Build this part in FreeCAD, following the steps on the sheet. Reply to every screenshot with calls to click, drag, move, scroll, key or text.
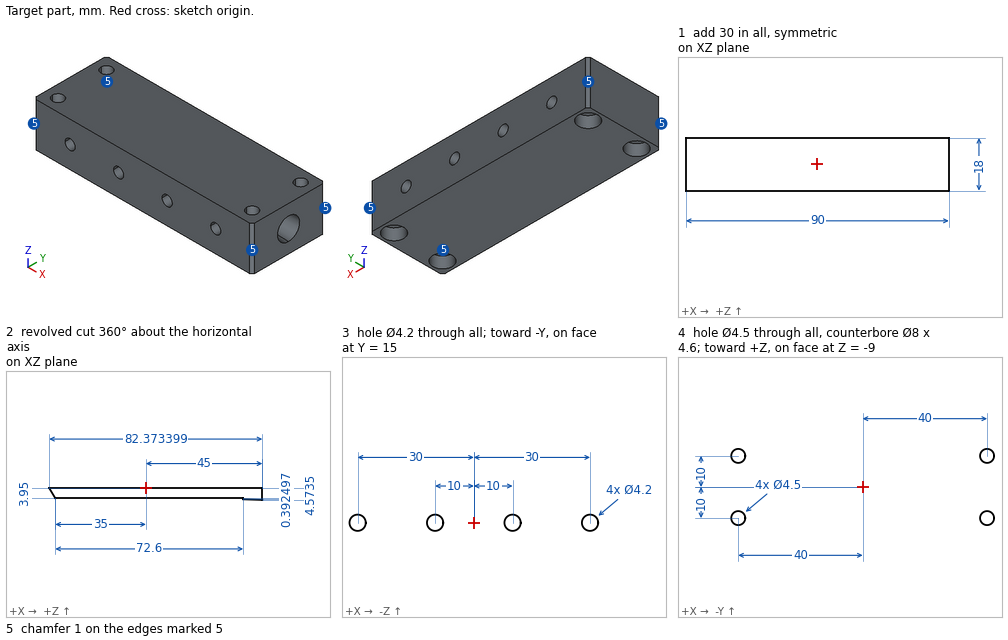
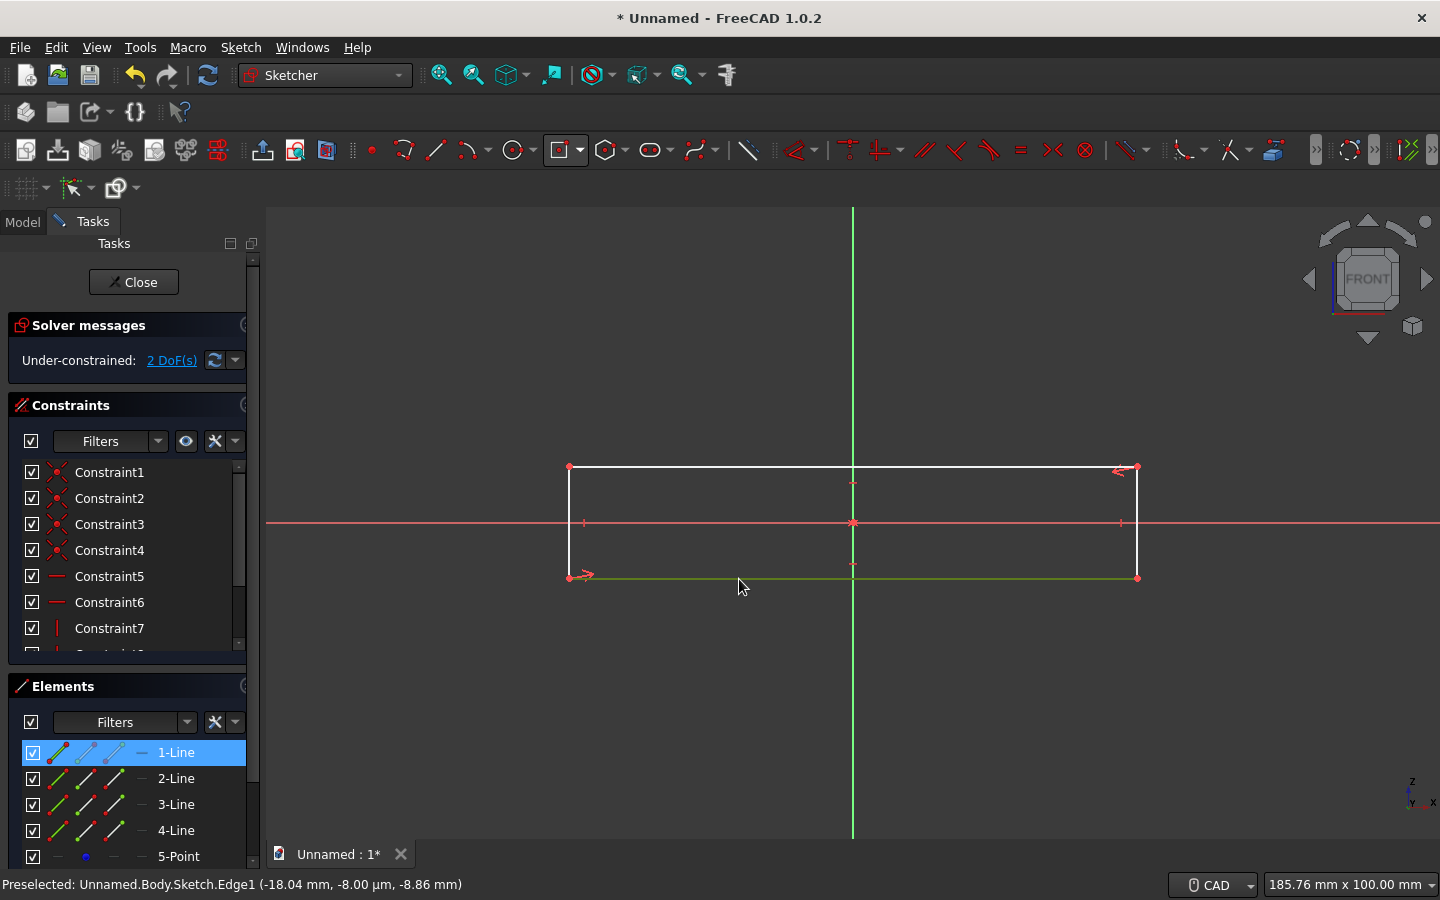
click(816, 150)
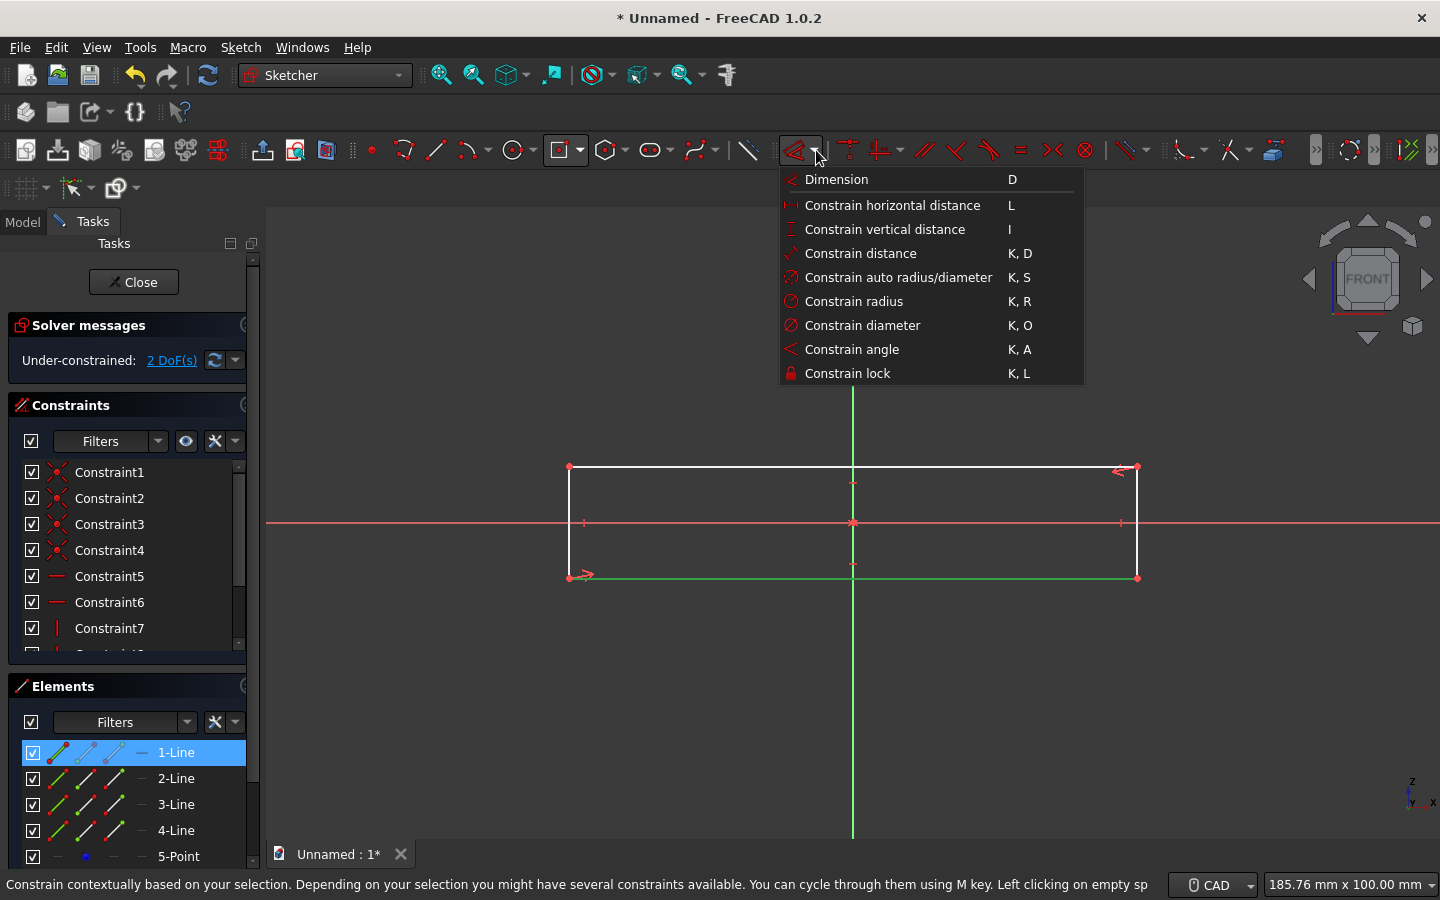
click(932, 205)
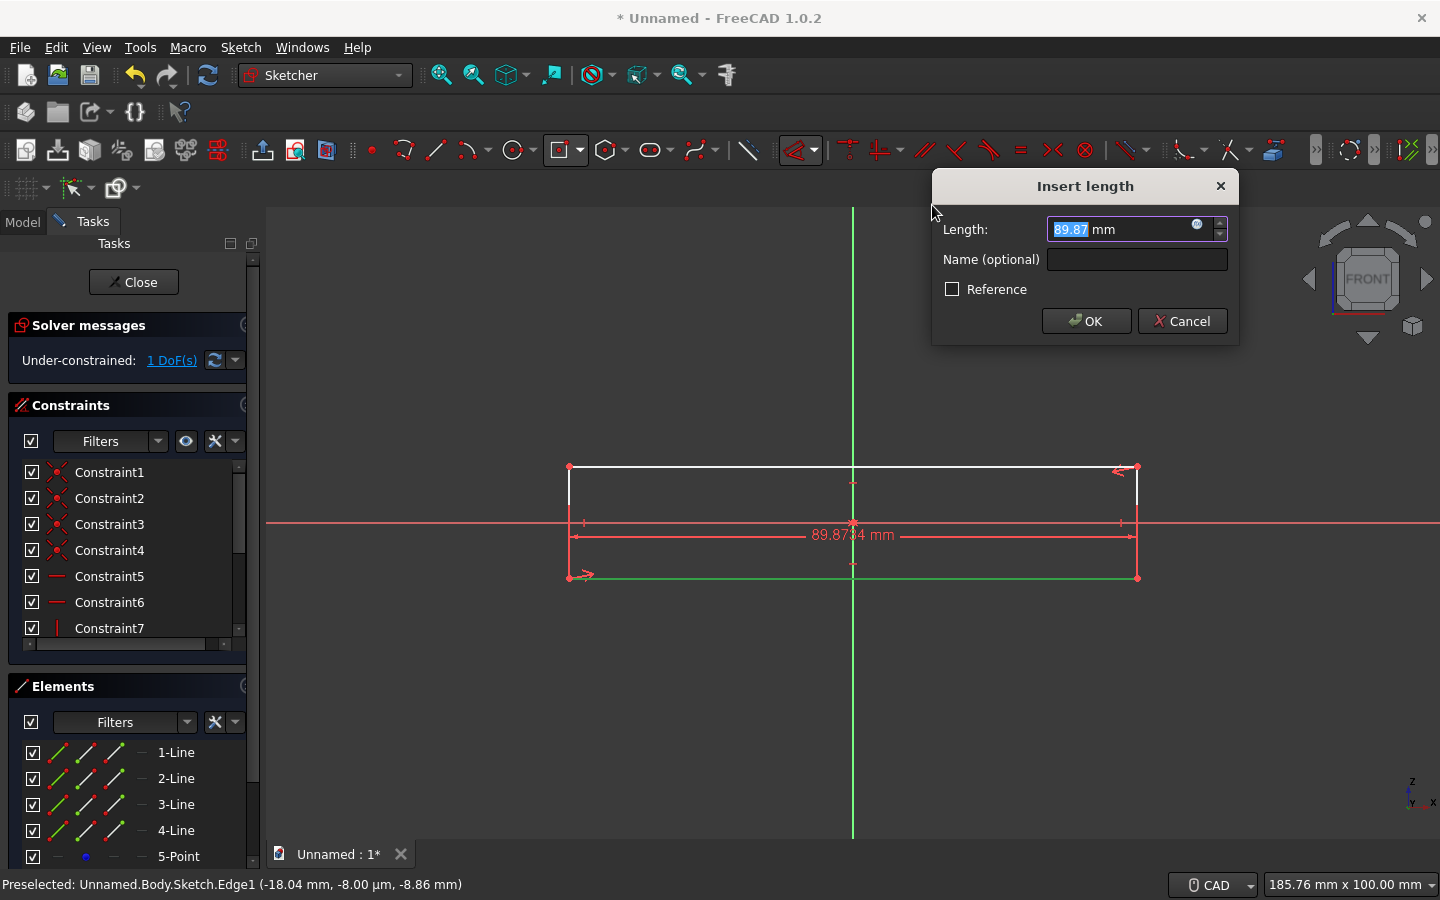
text(90)
key(Return)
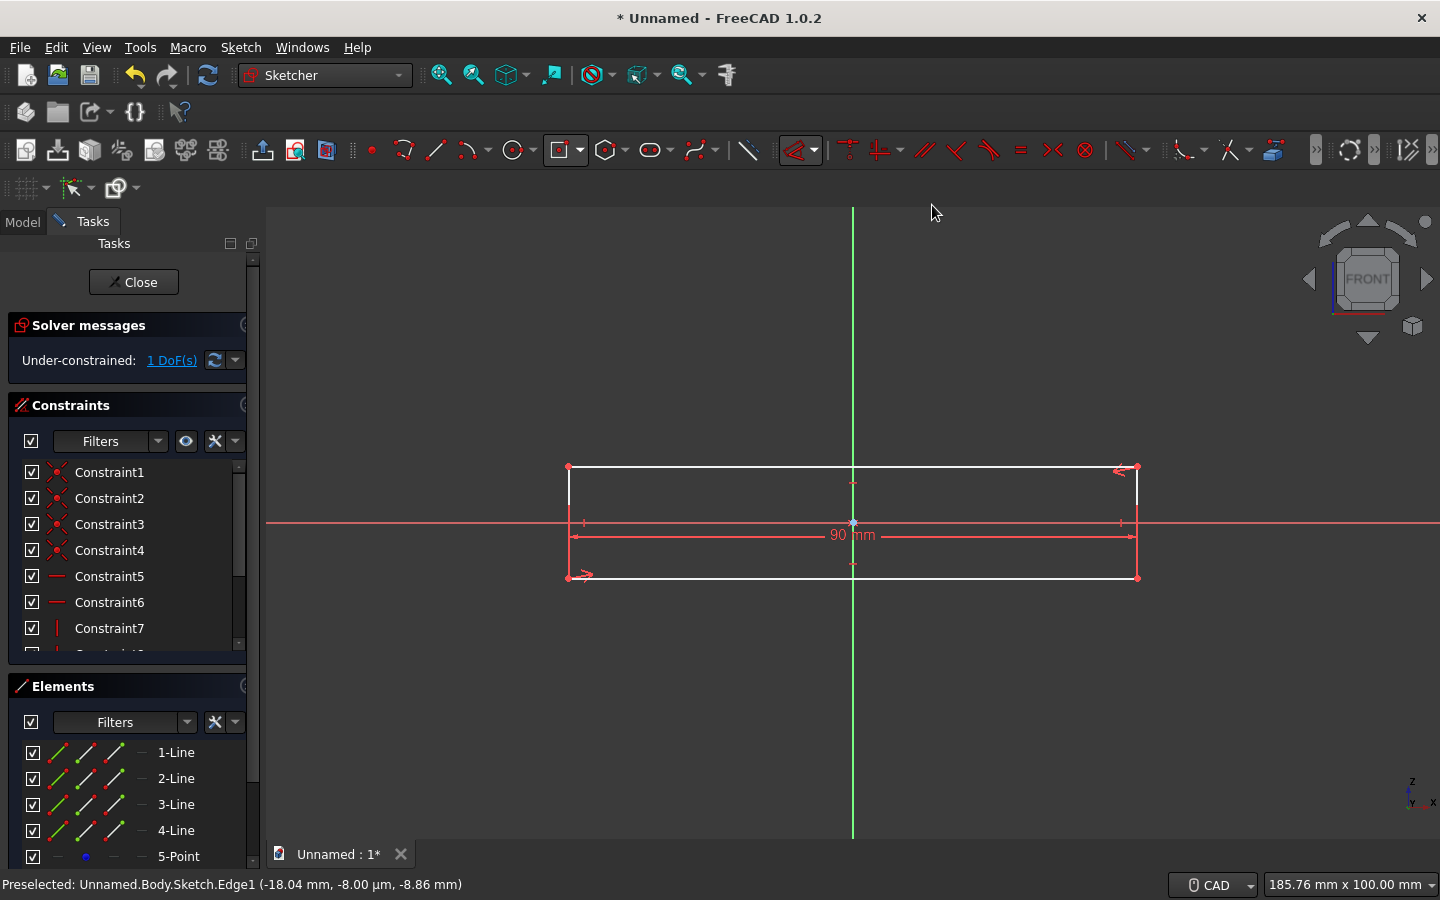
click(1137, 545)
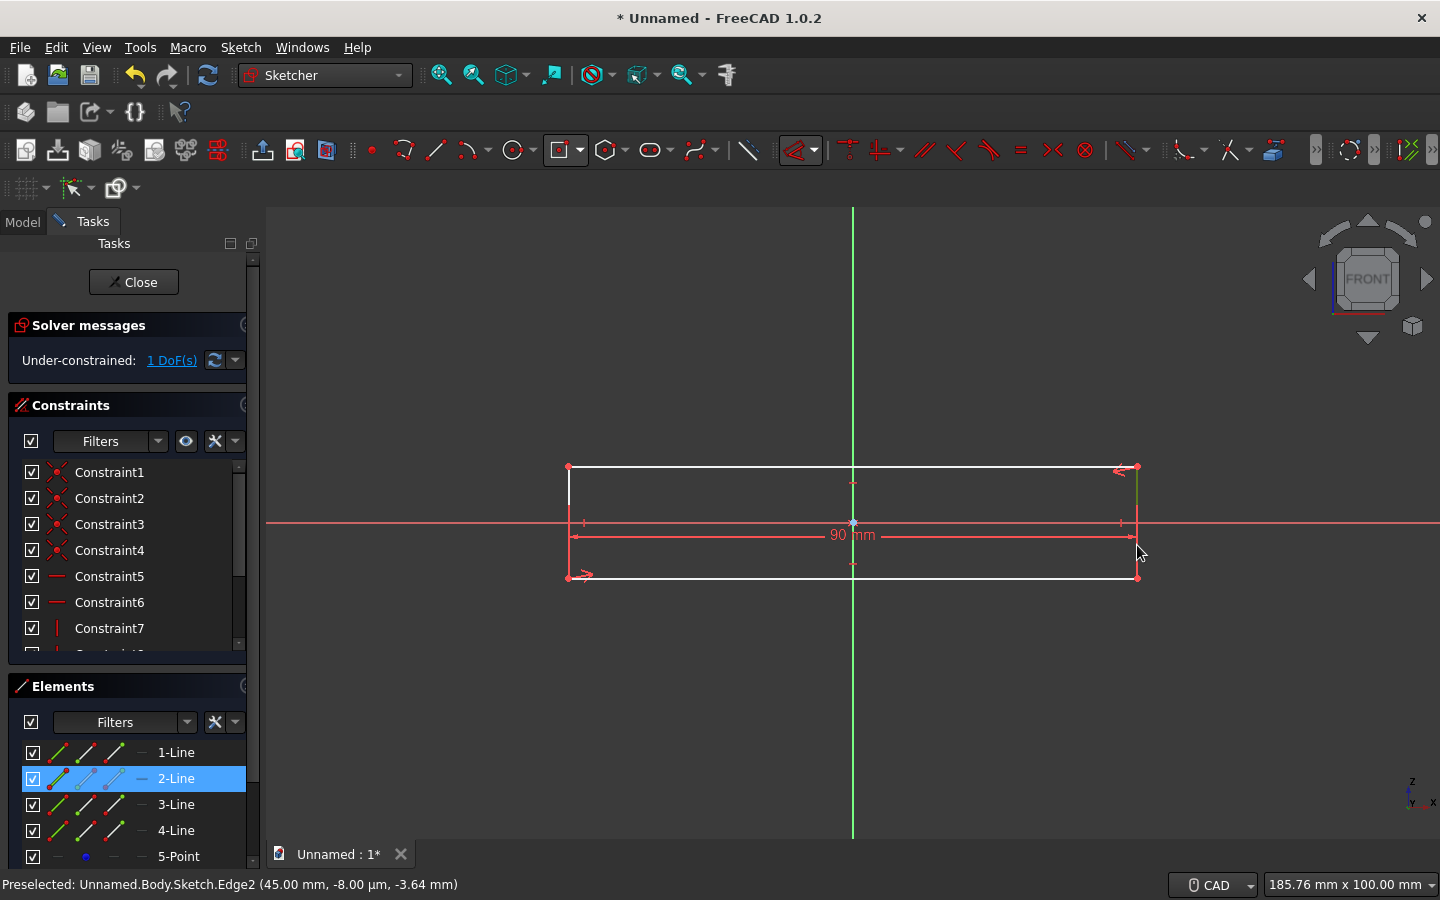
click(816, 150)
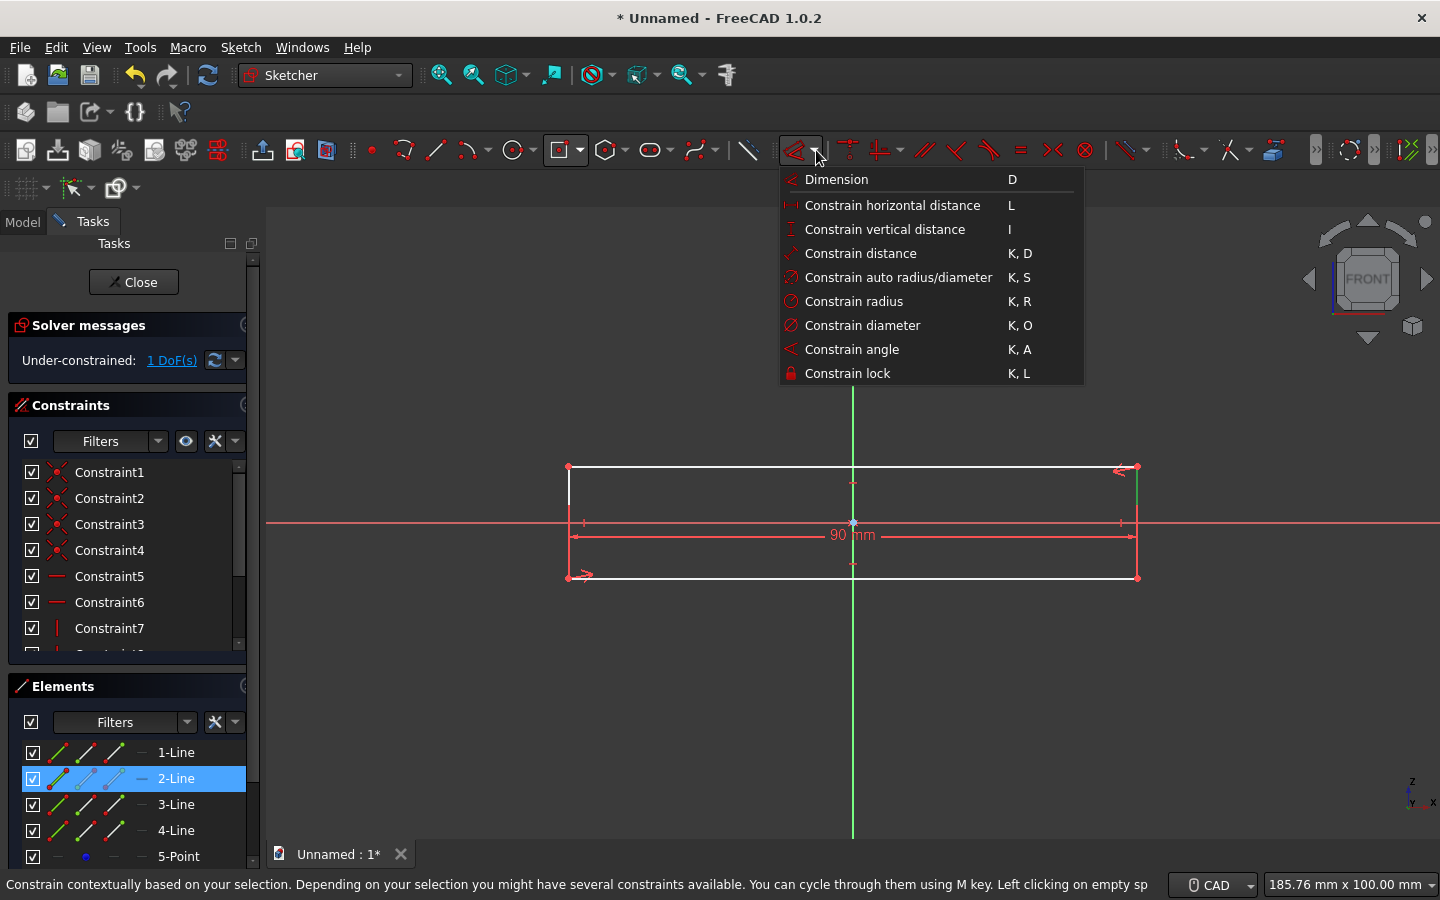
click(932, 229)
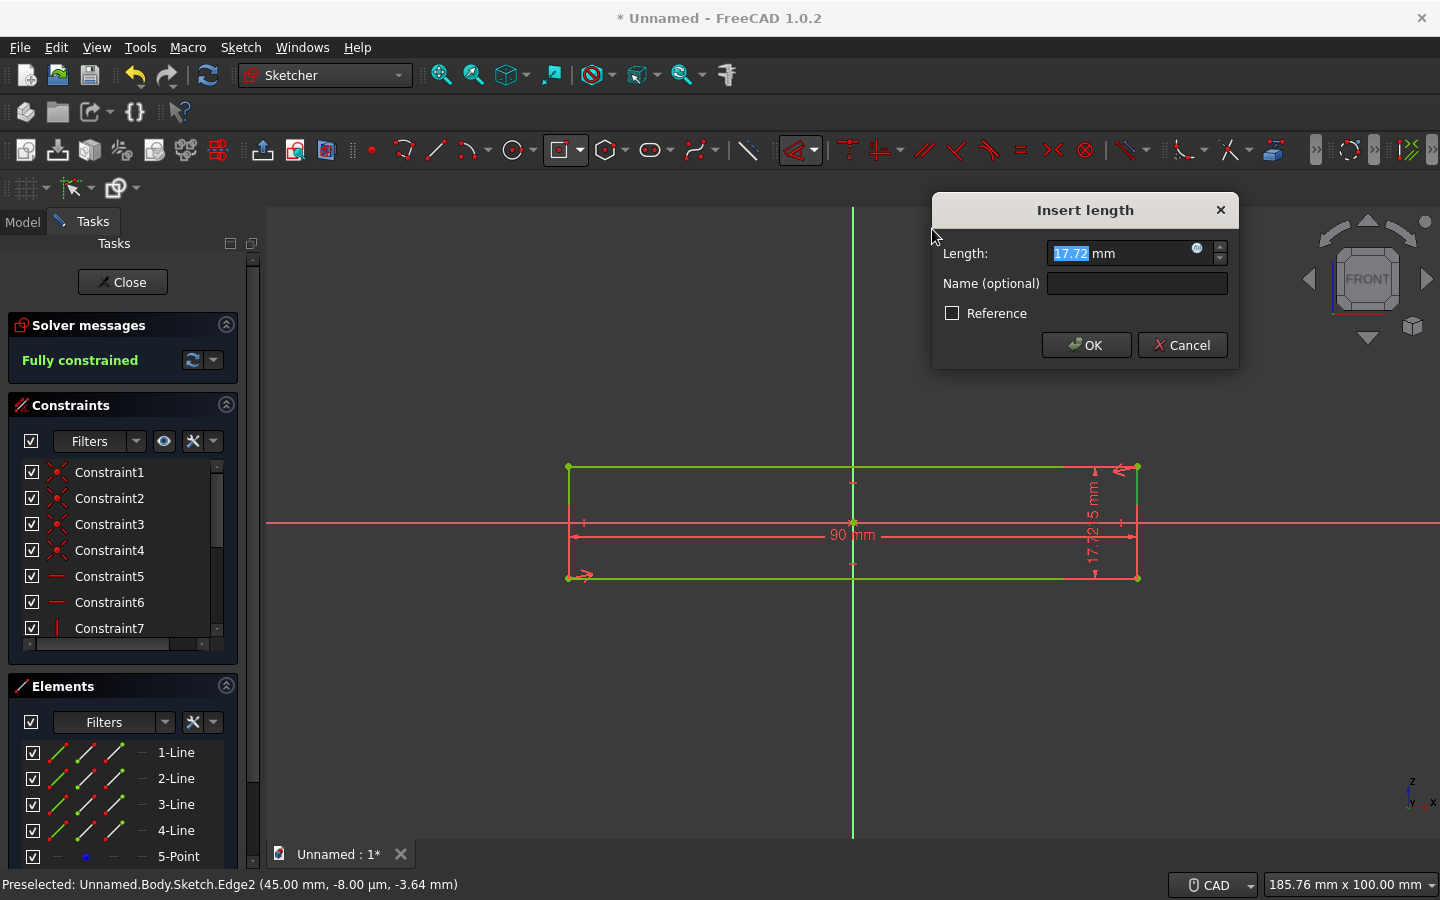
text(18)
key(Return)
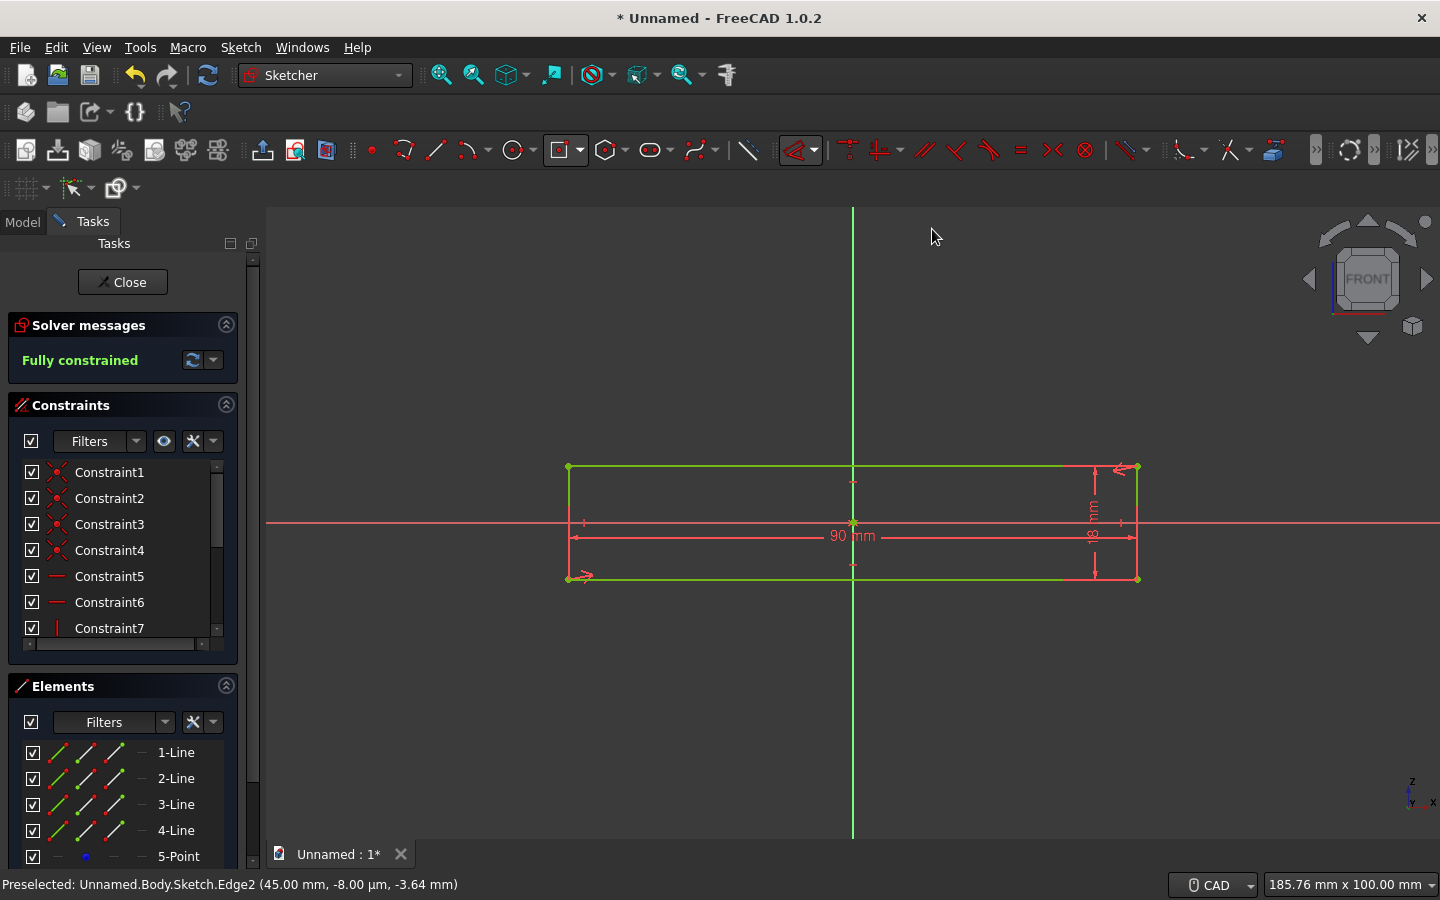
click(123, 282)